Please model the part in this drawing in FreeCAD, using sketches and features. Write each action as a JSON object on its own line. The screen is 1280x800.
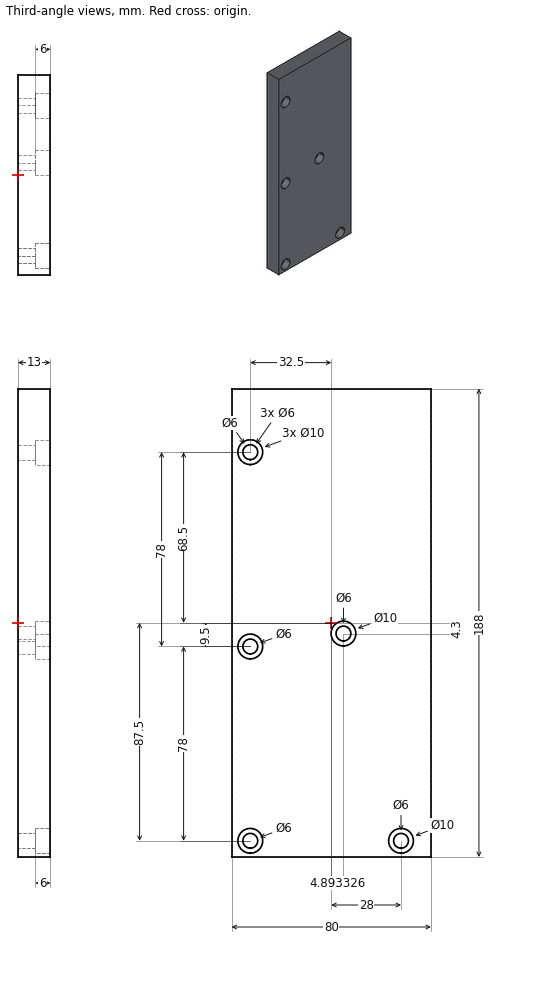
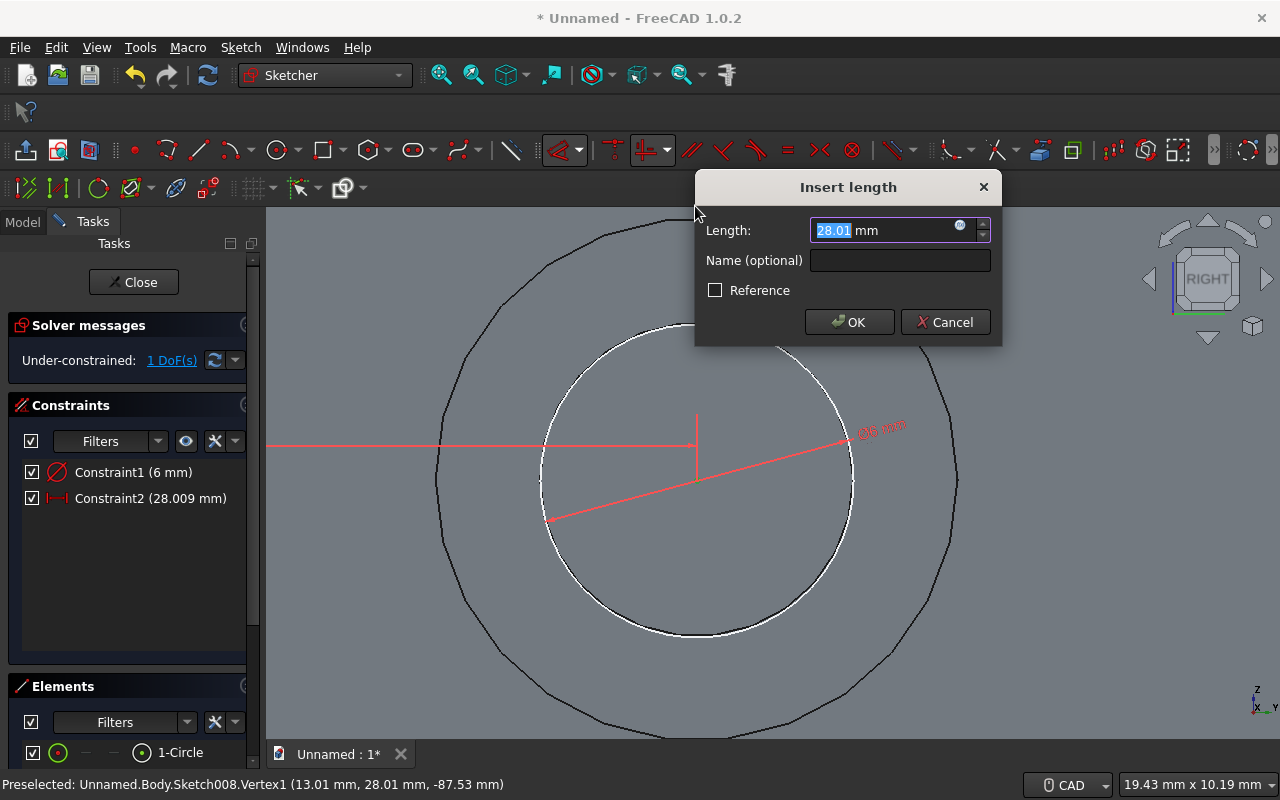
{"action": "type", "text": "28"}
{"action": "key", "text": "Return"}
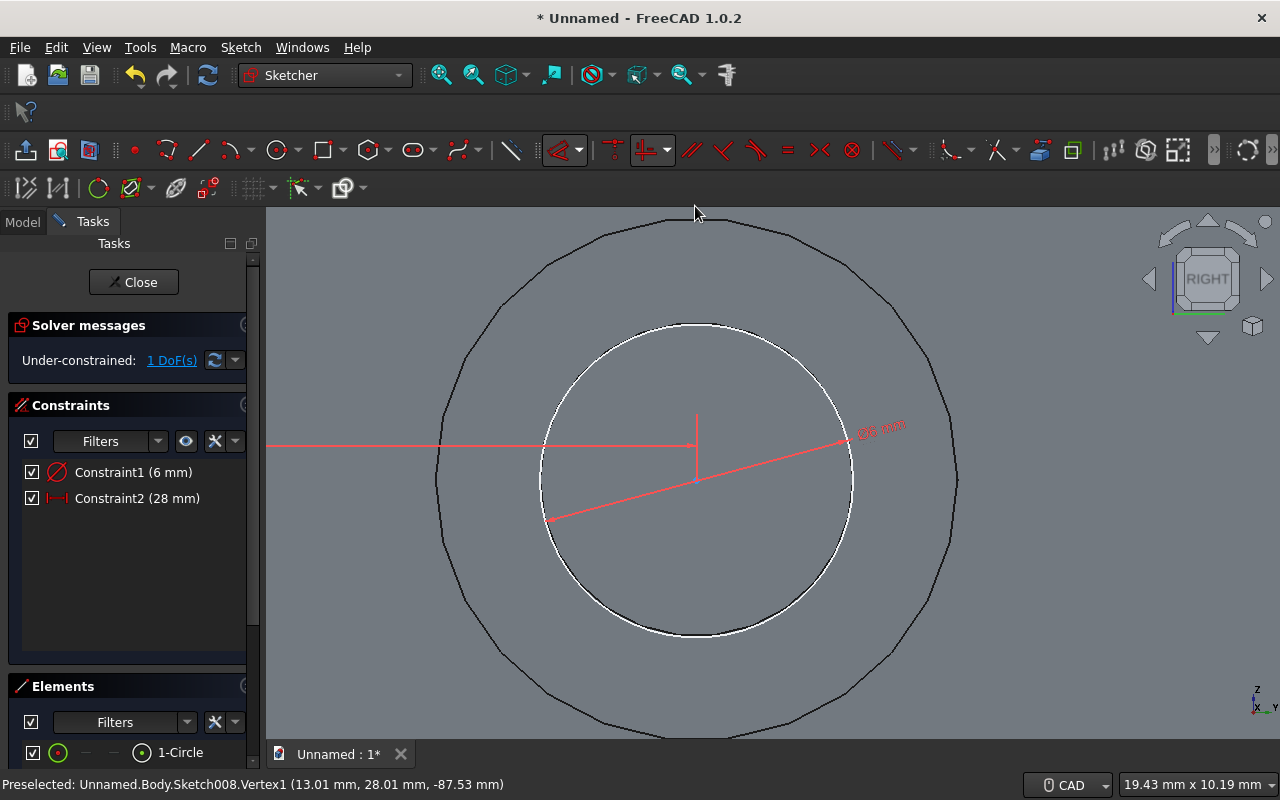
{"action": "left_click", "coordinate": [697, 481]}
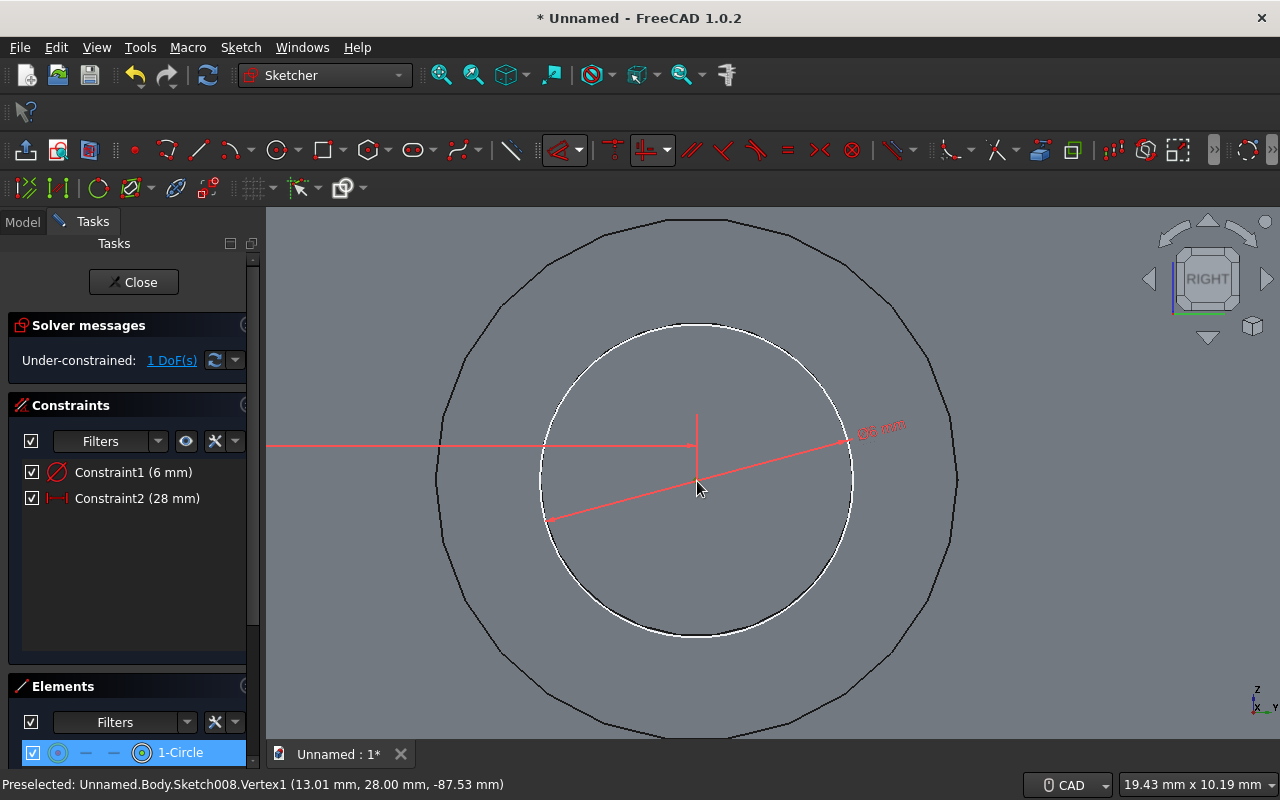
{"action": "key", "text": "i"}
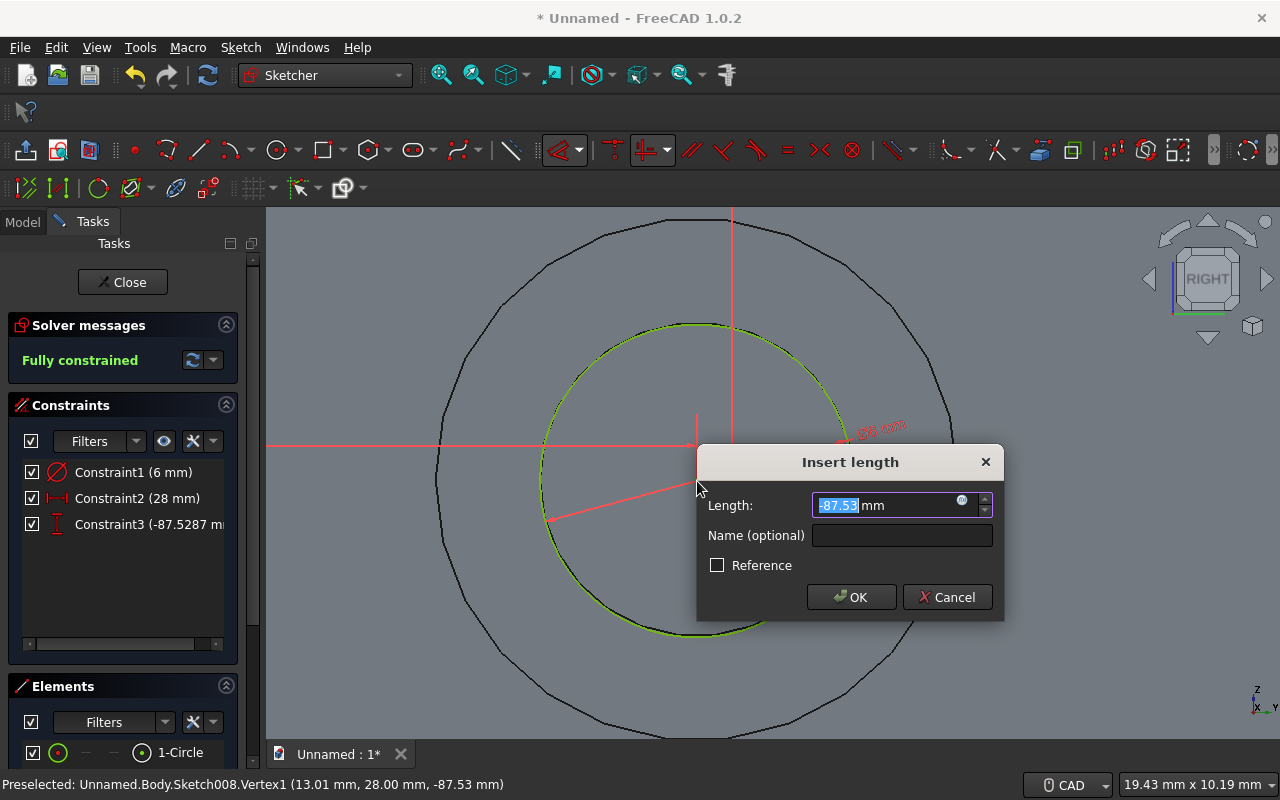
{"action": "type", "text": "-87.5"}
{"action": "key", "text": "Return"}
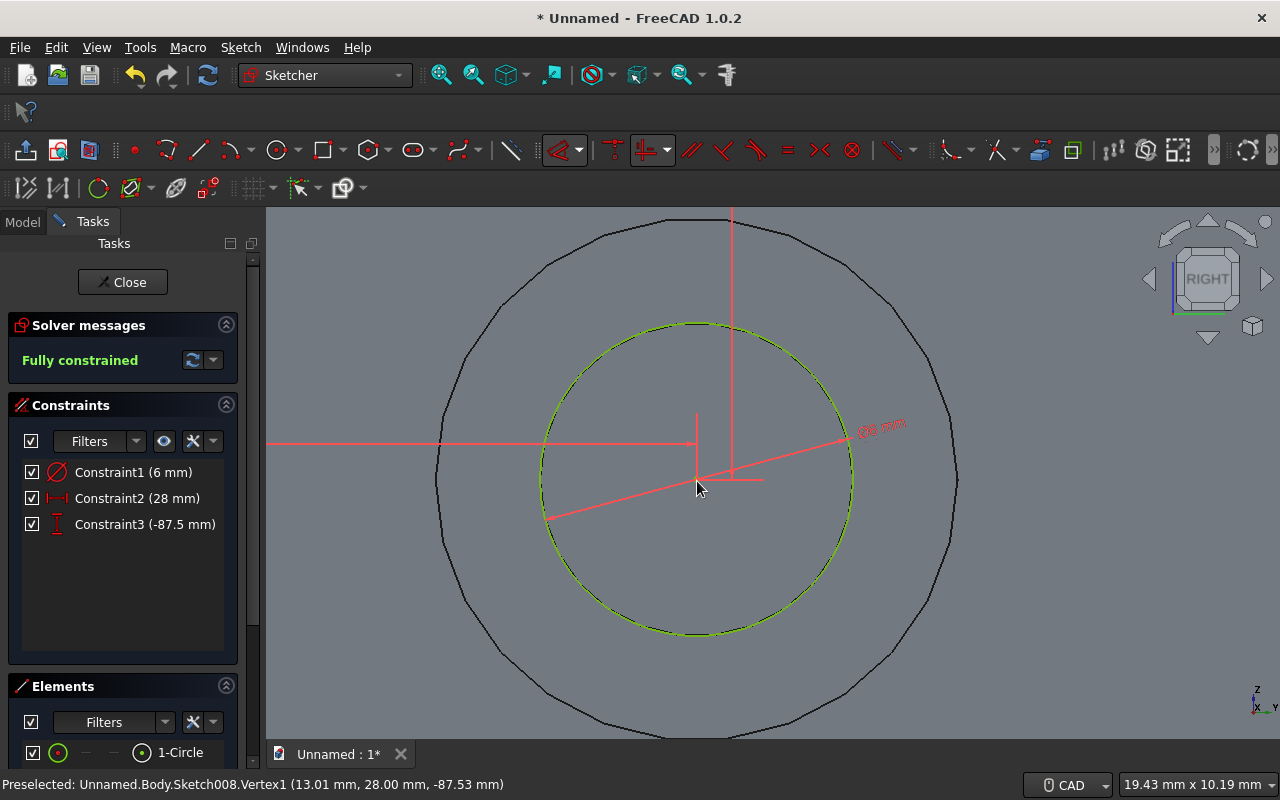
{"action": "left_click", "coordinate": [123, 282]}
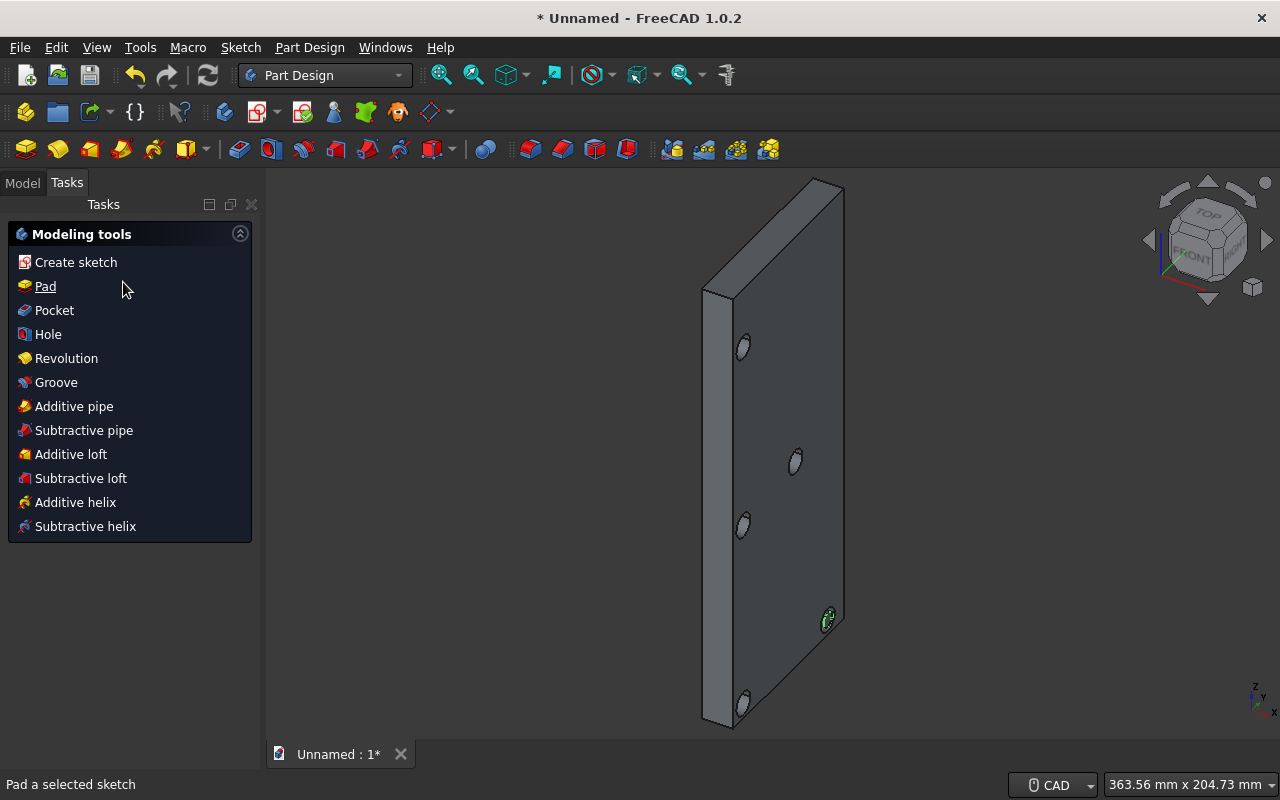
{"action": "left_click", "coordinate": [240, 150]}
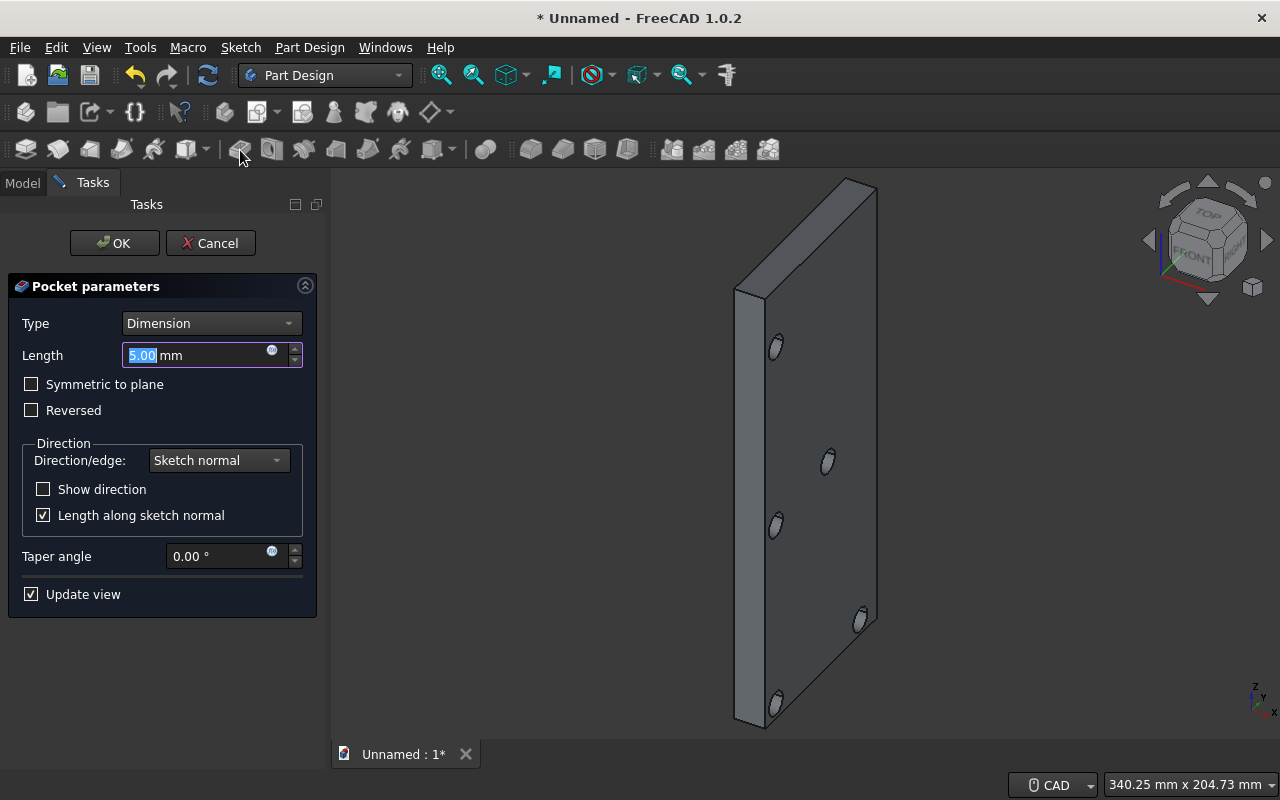
{"action": "left_click", "coordinate": [212, 324]}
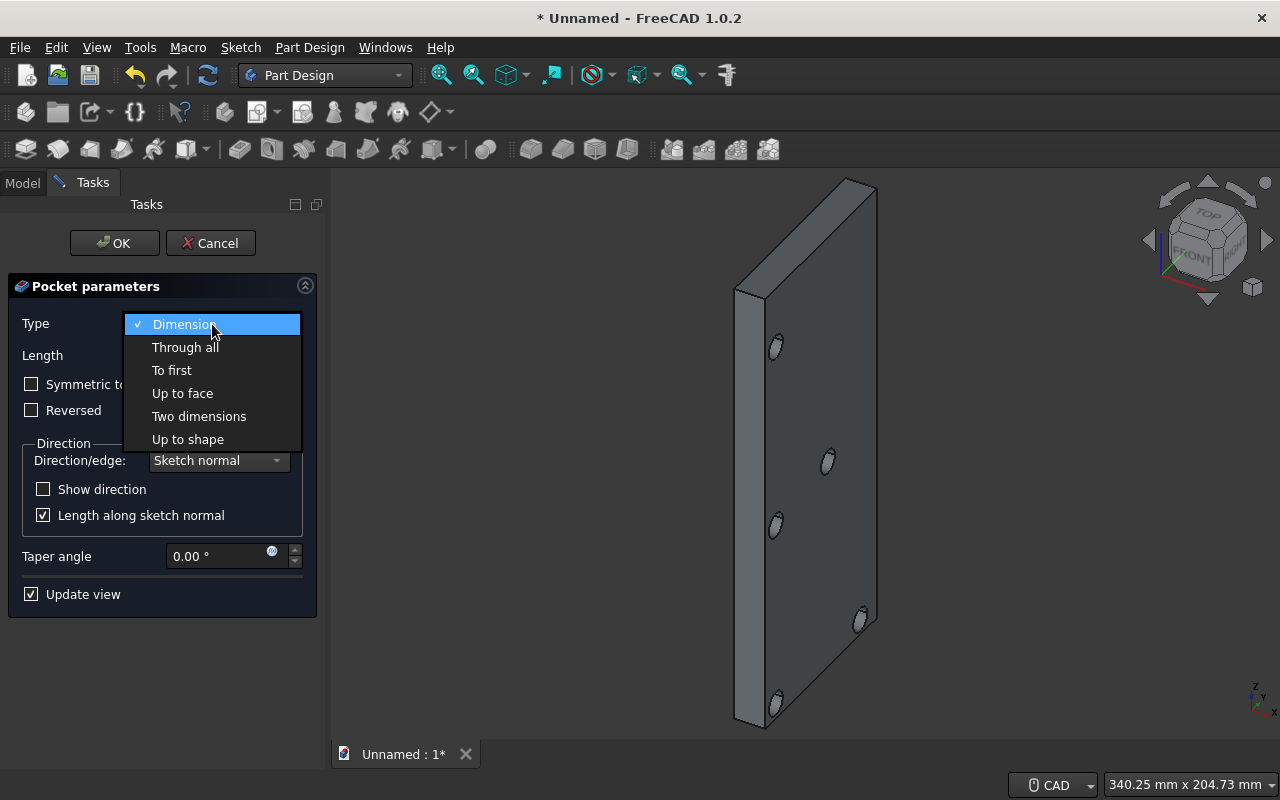
{"action": "left_click", "coordinate": [212, 370]}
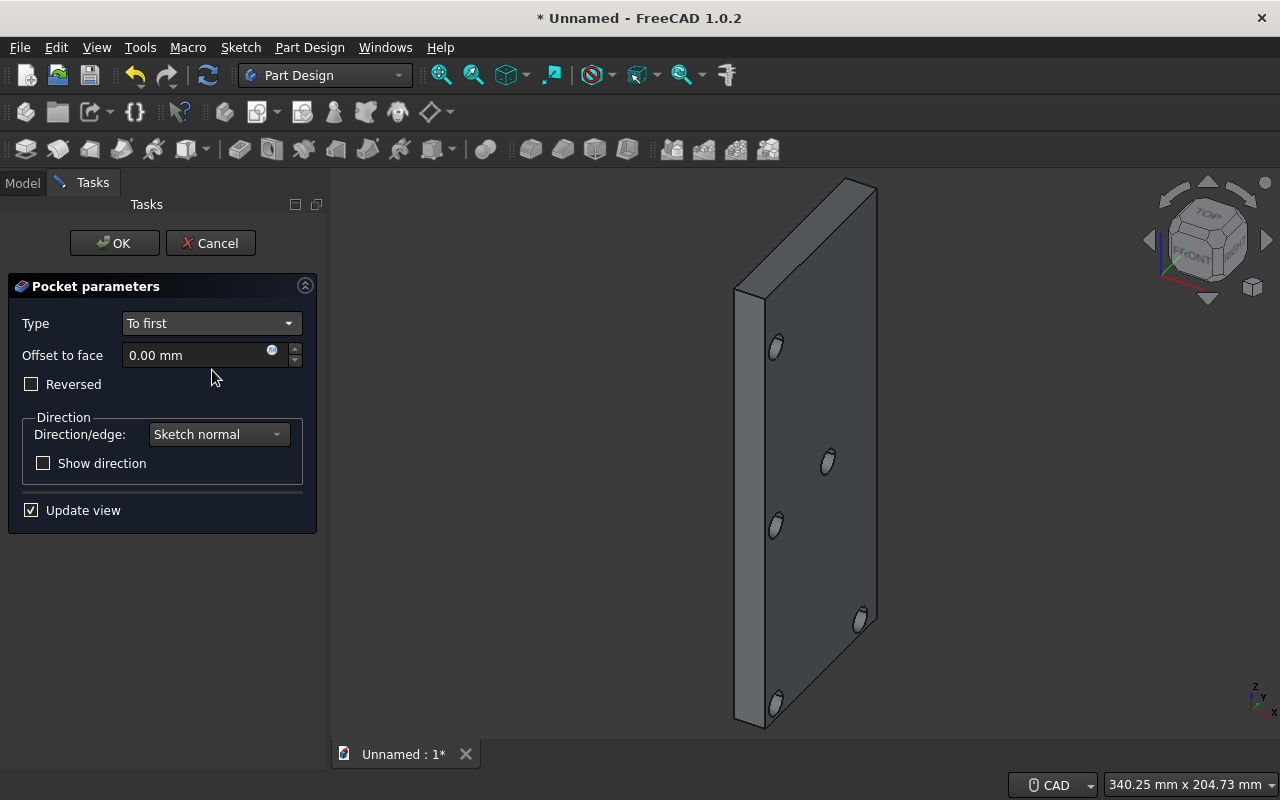
{"action": "left_click", "coordinate": [115, 243]}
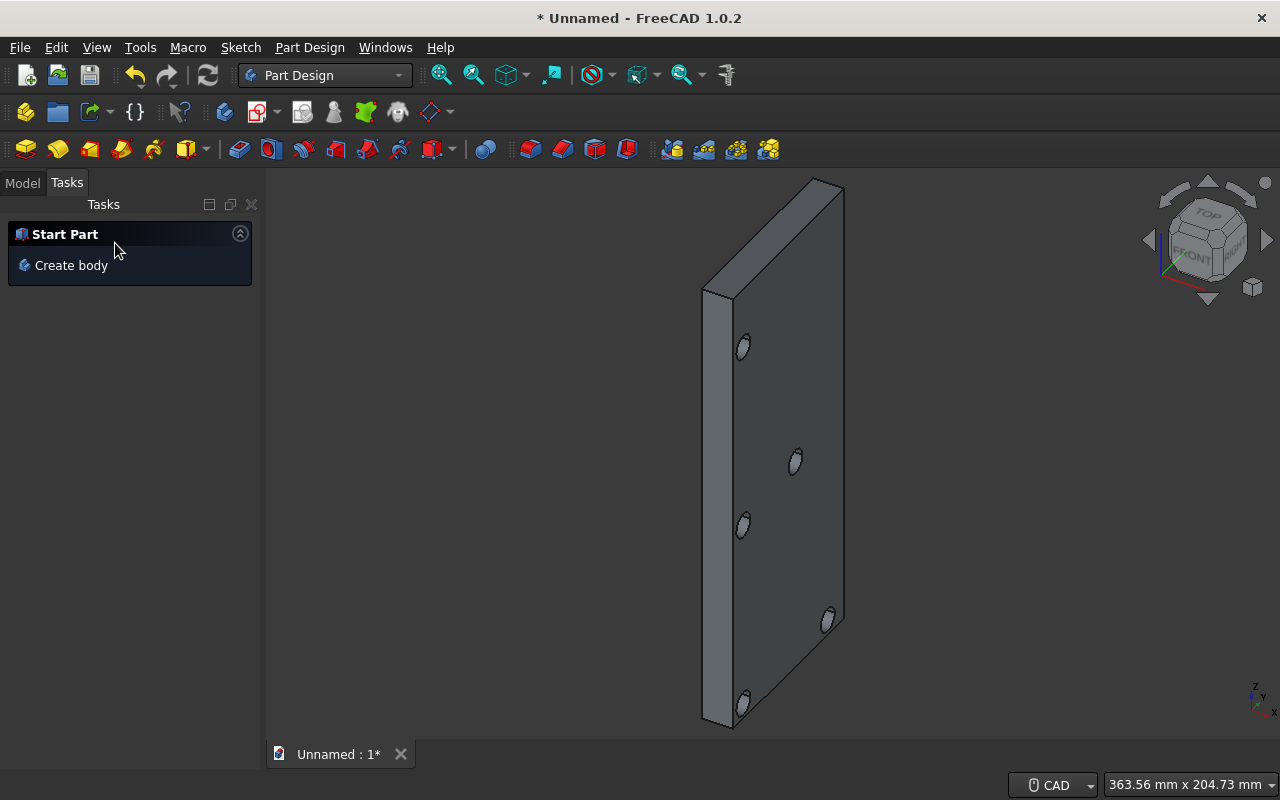
{"action": "key", "text": "0"}